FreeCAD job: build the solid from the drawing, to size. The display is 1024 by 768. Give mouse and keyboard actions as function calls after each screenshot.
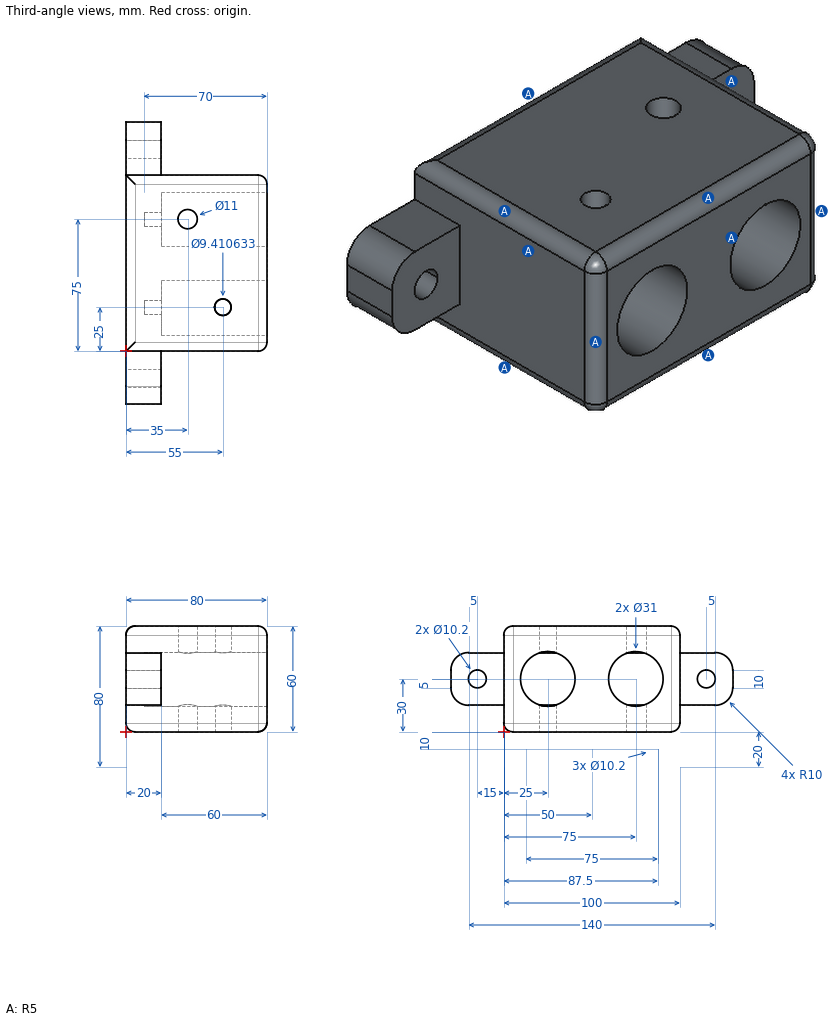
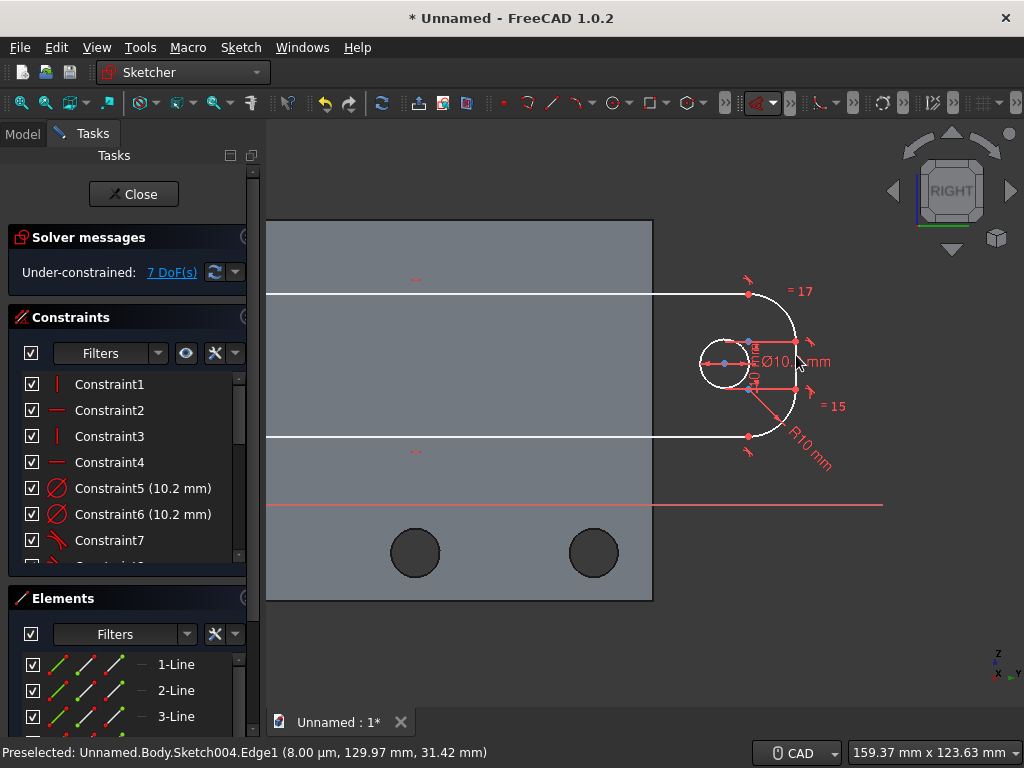
scroll(772, 431, down, 3)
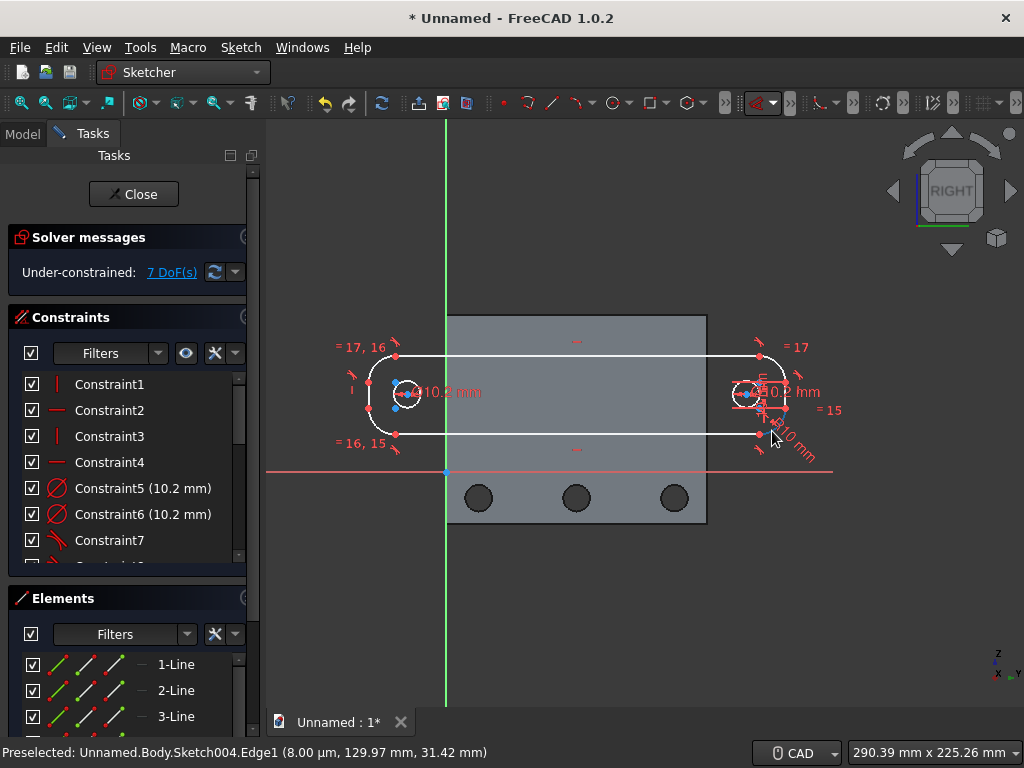
click(407, 394)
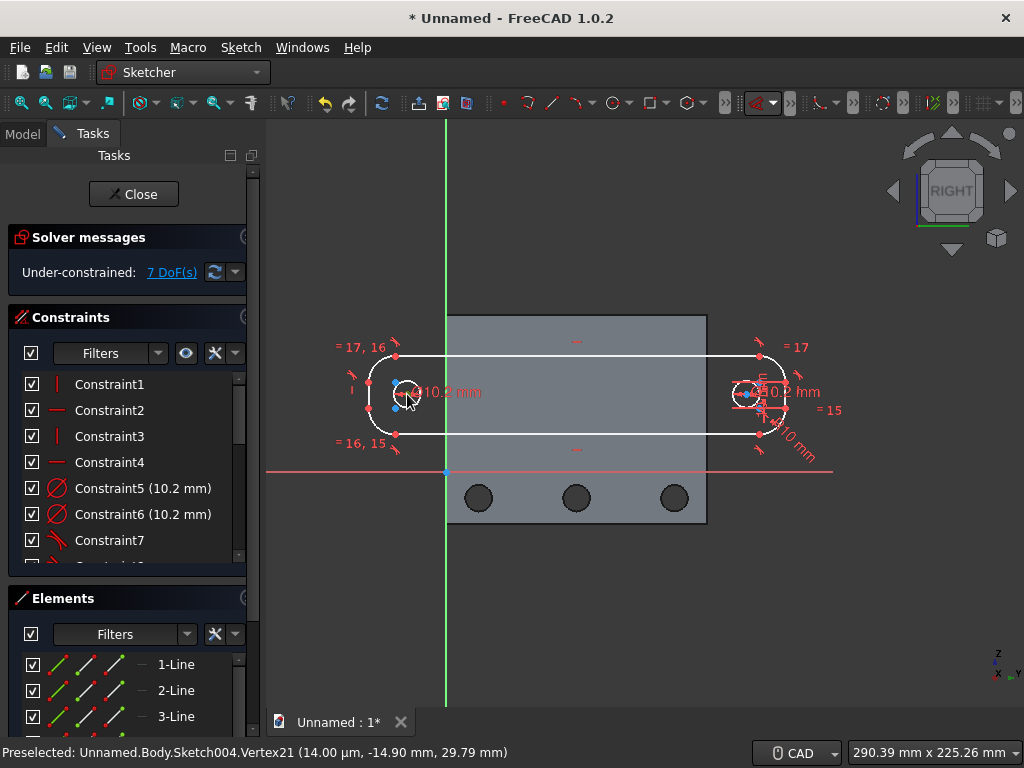
click(776, 104)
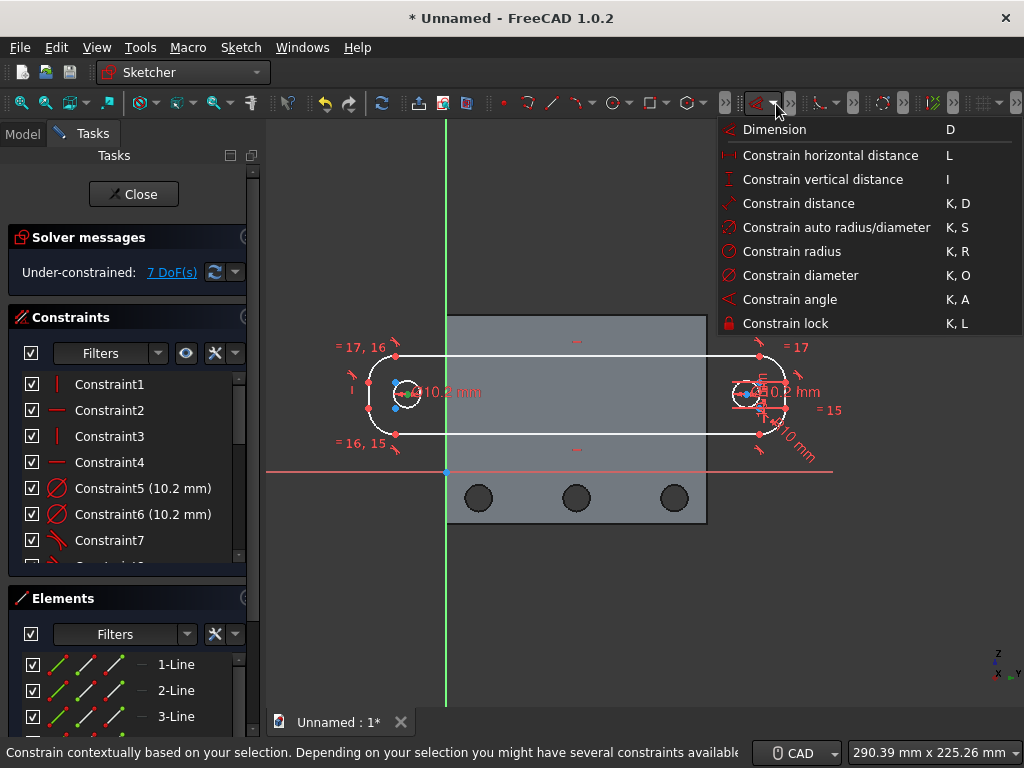
click(870, 155)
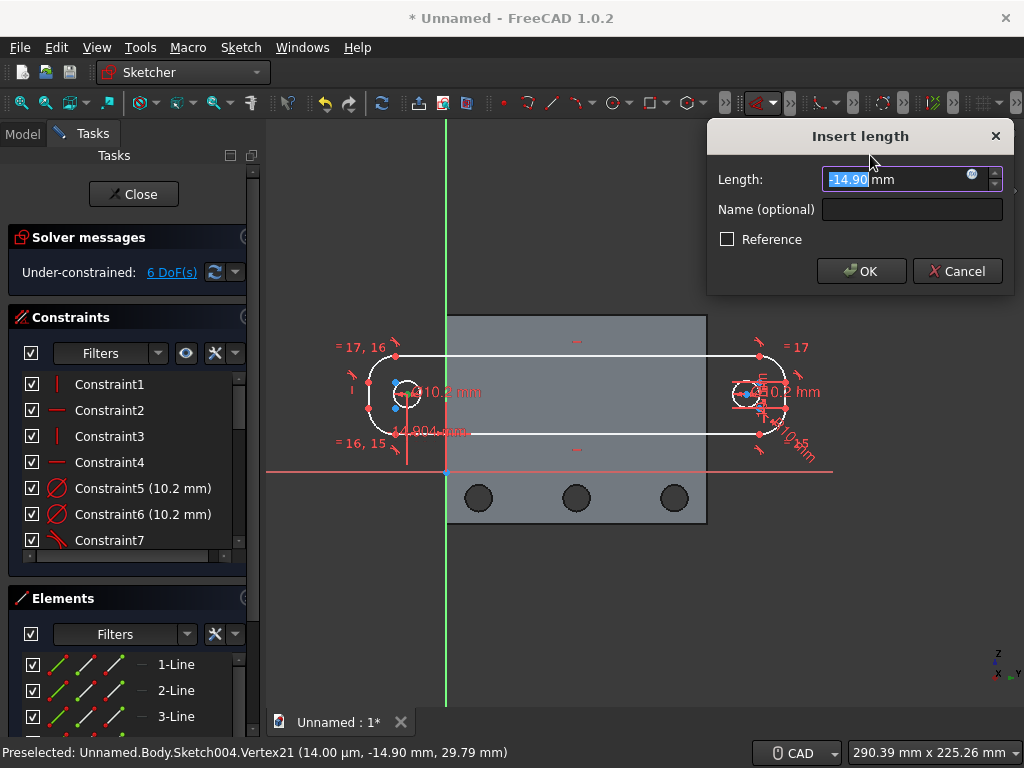
text(-15)
key(Return)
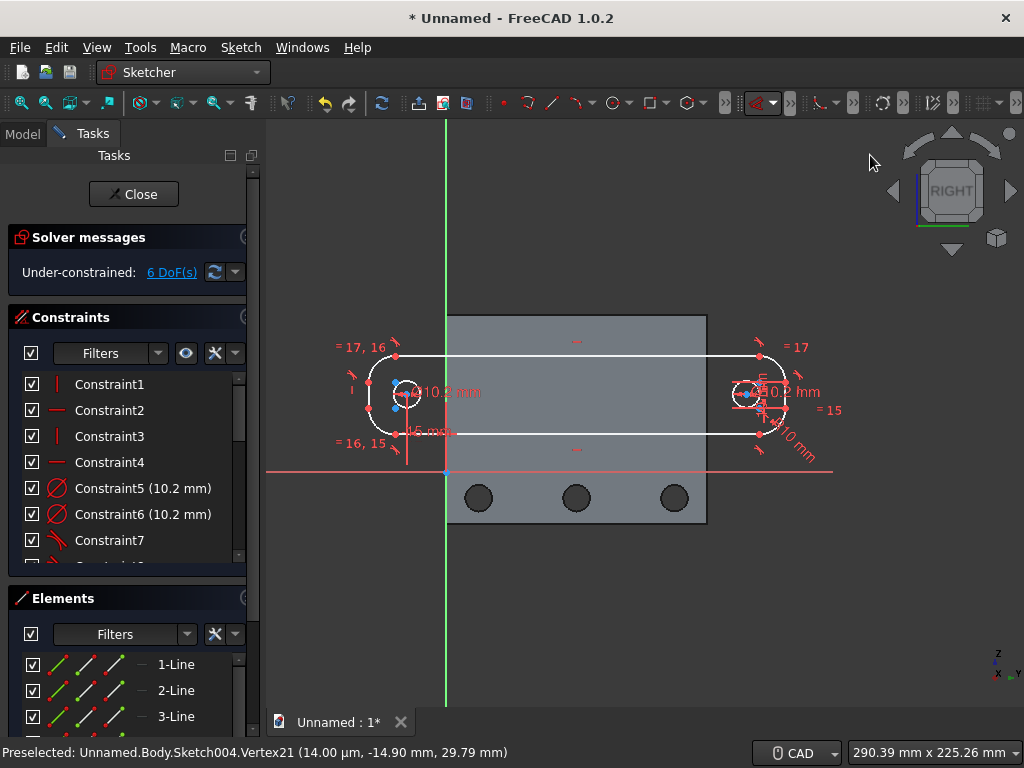
click(407, 394)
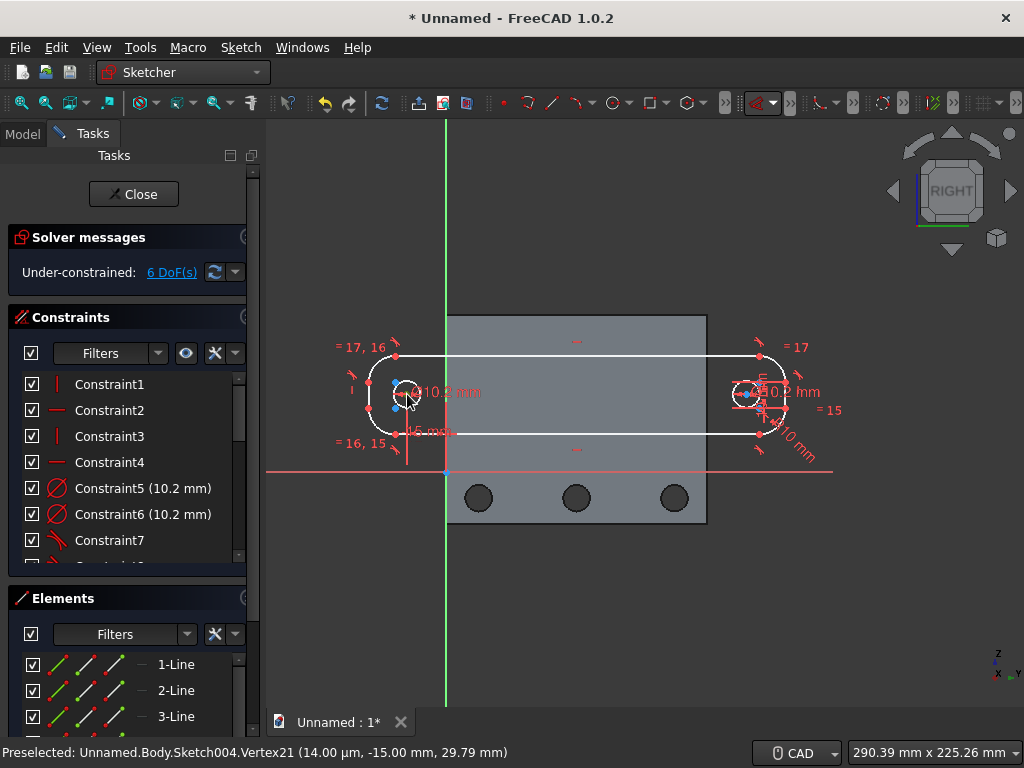
click(776, 104)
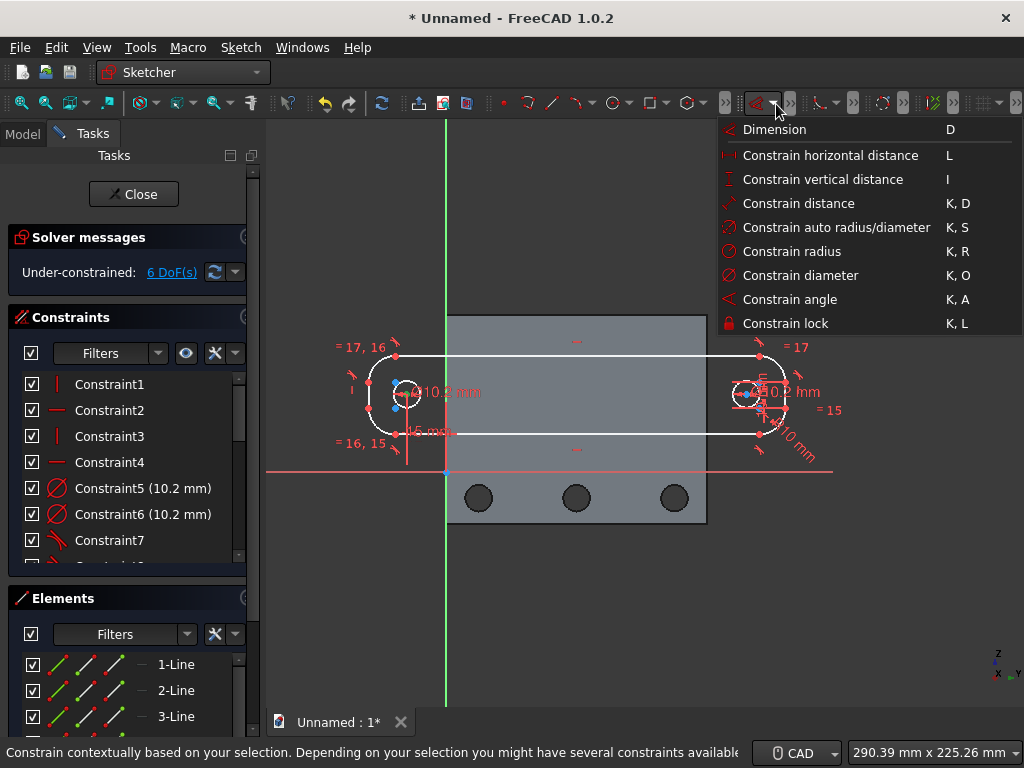
click(870, 179)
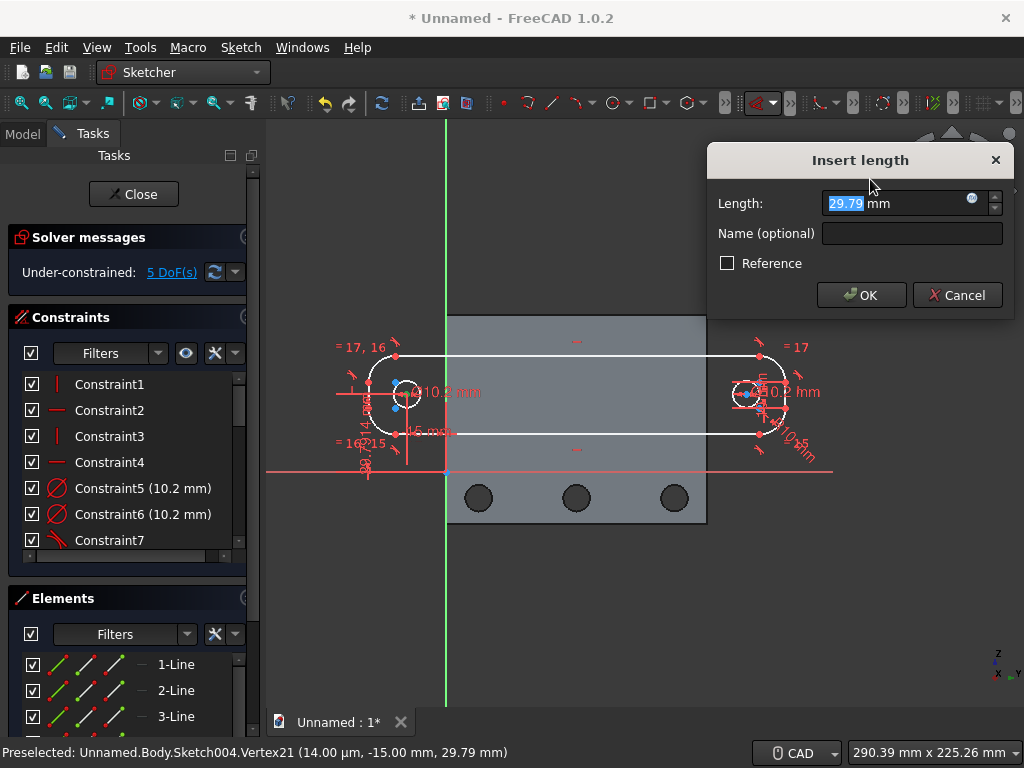
text(30)
key(Return)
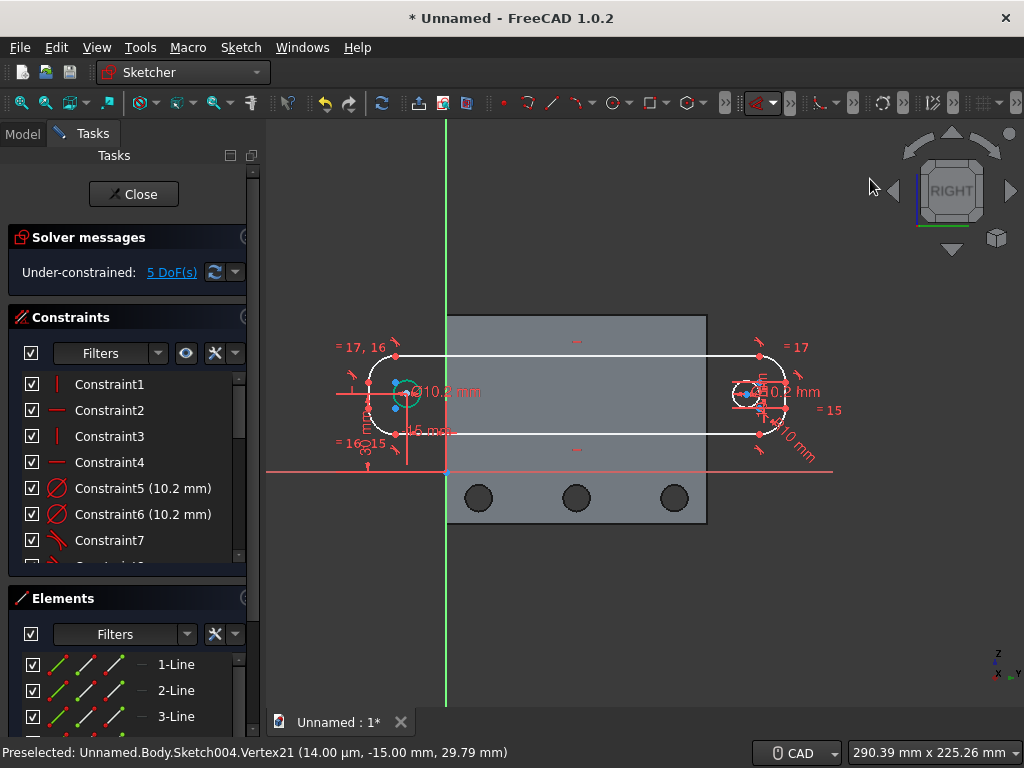
click(746, 394)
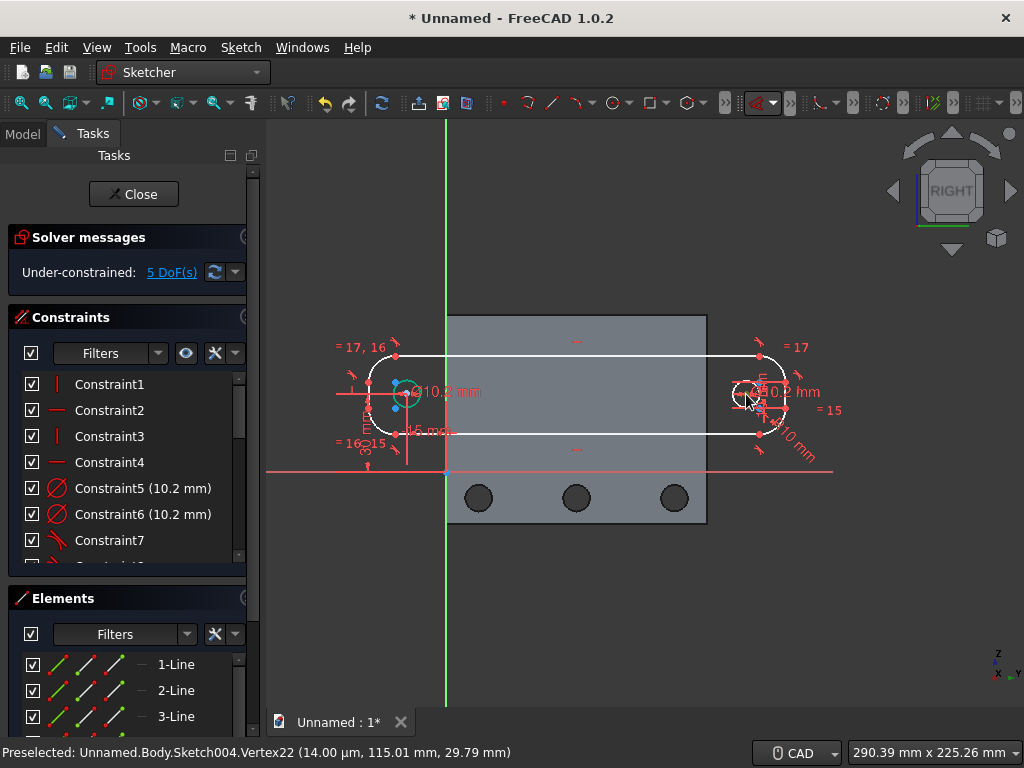
key(i)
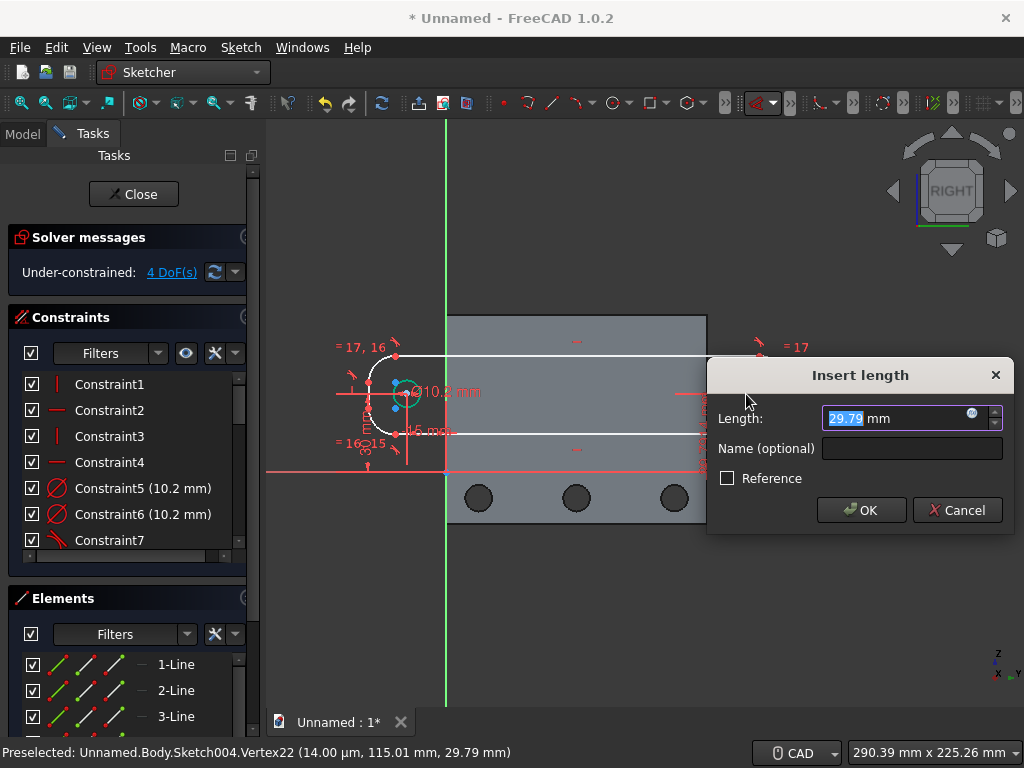
text(30)
key(Return)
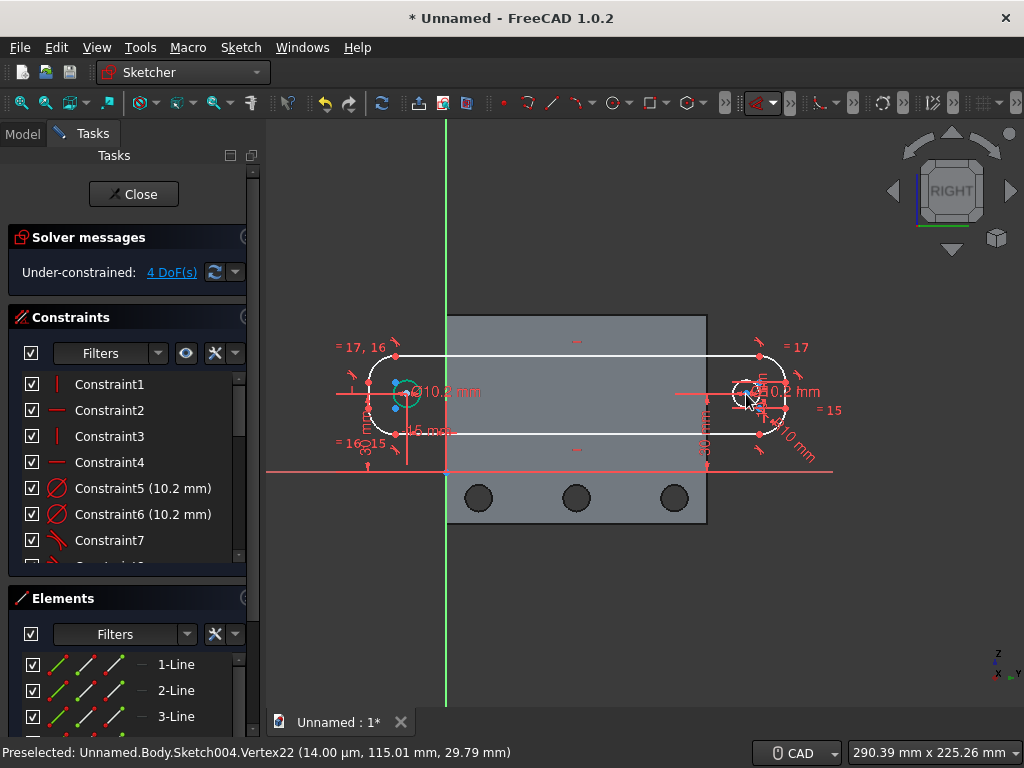
scroll(395, 434, up, 6)